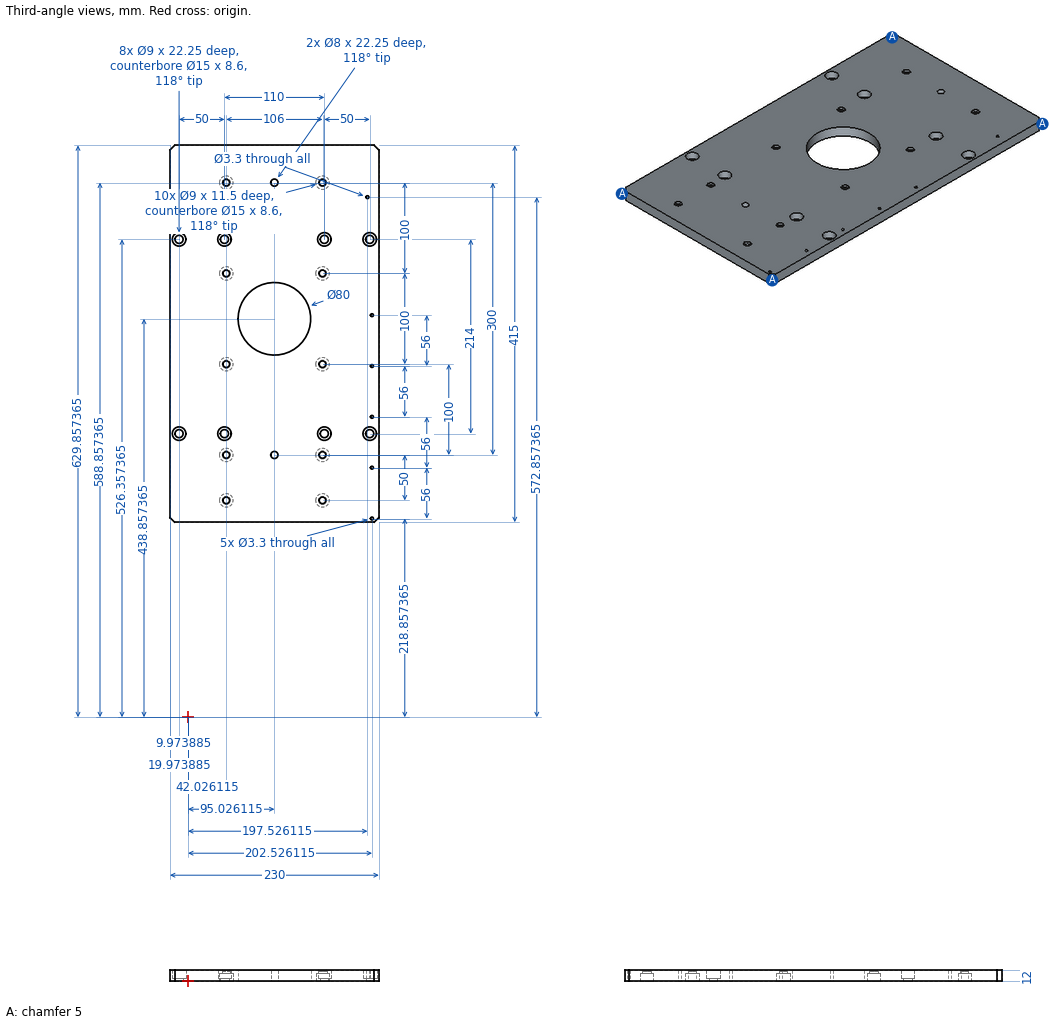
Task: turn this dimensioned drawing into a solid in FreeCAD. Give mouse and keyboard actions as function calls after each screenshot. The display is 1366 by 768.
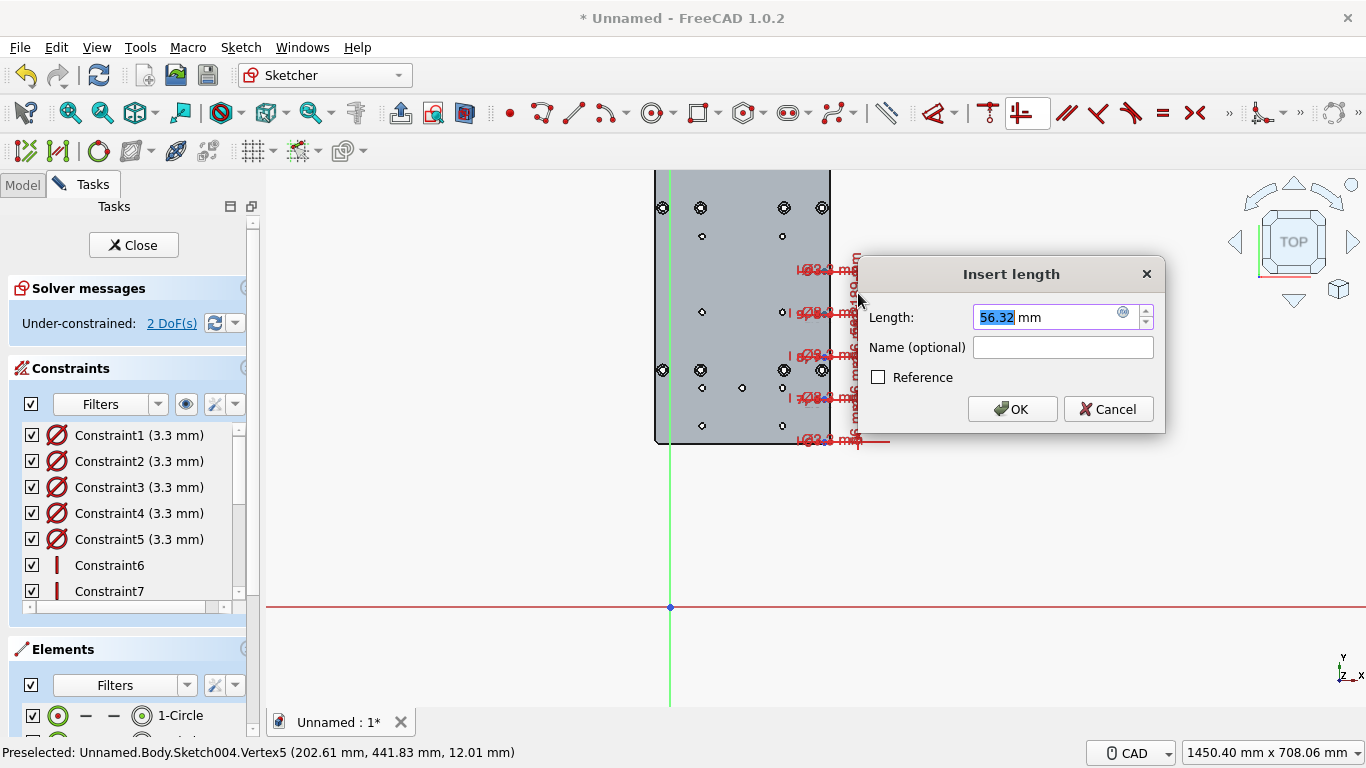
text(56)
key(Return)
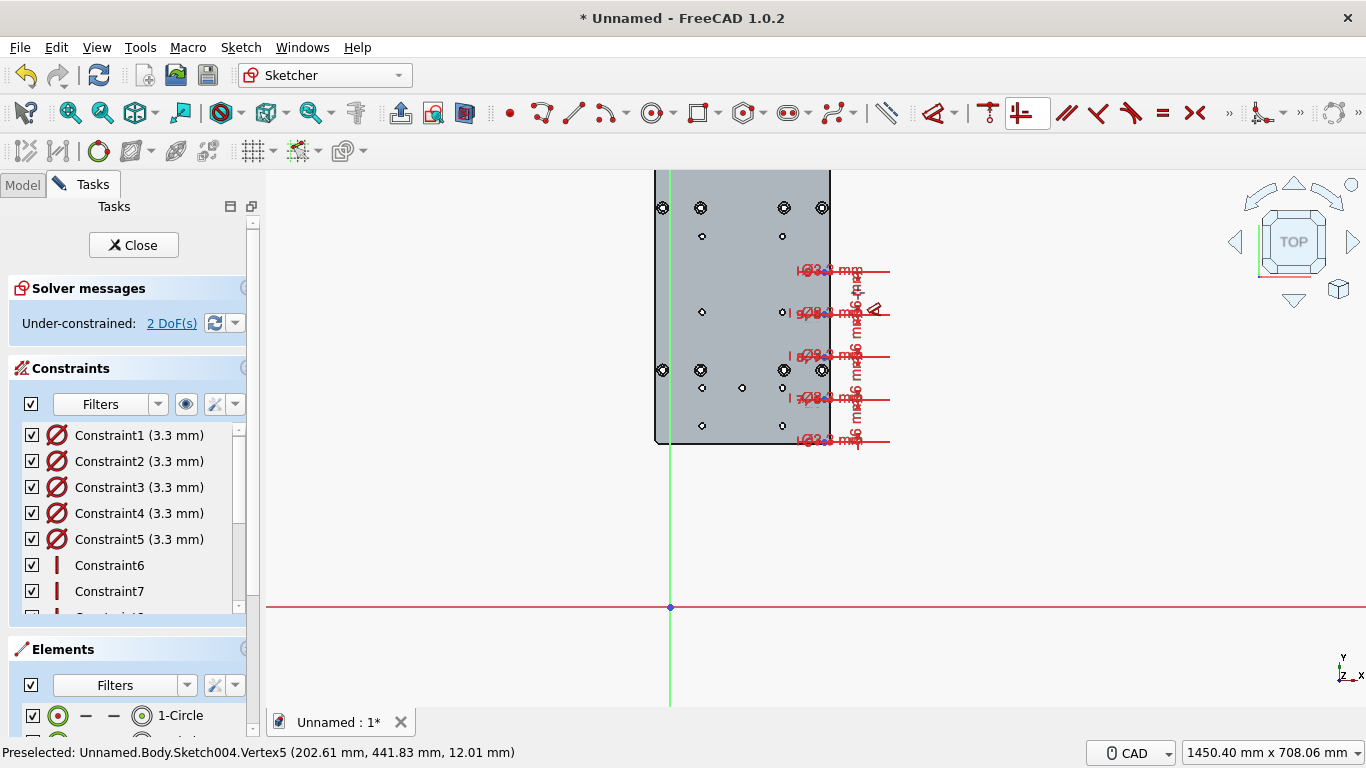
click(824, 442)
click(747, 641)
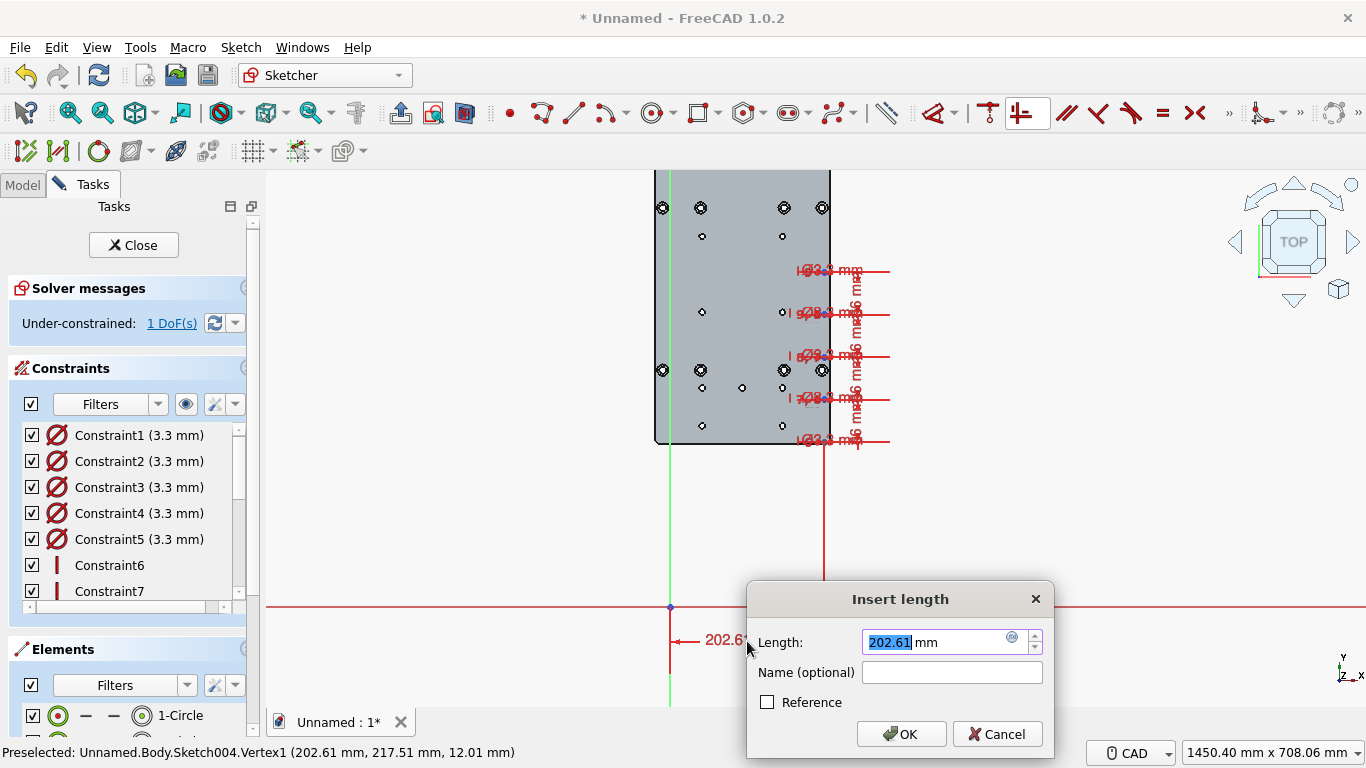
text(202.526115)
key(Return)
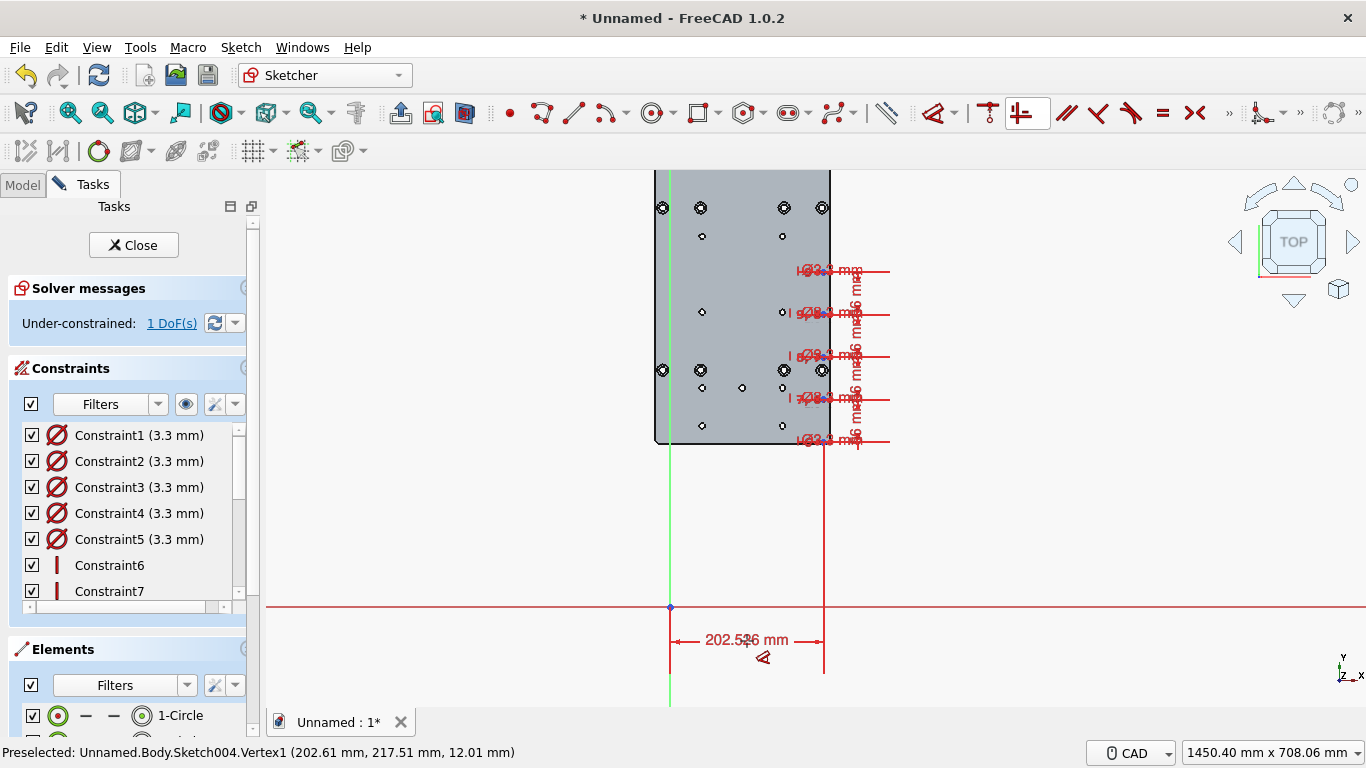
click(824, 442)
click(636, 525)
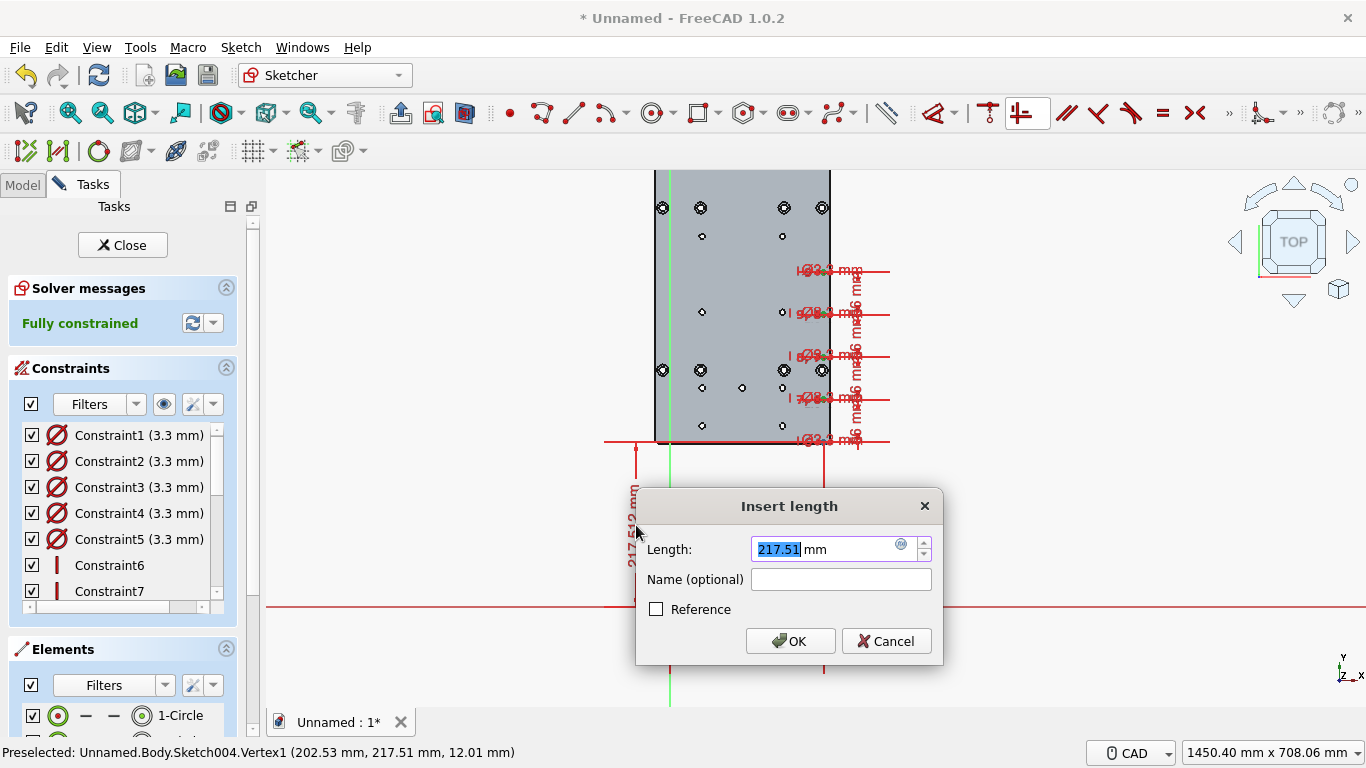
text(218.857365)
key(Return)
key(Escape)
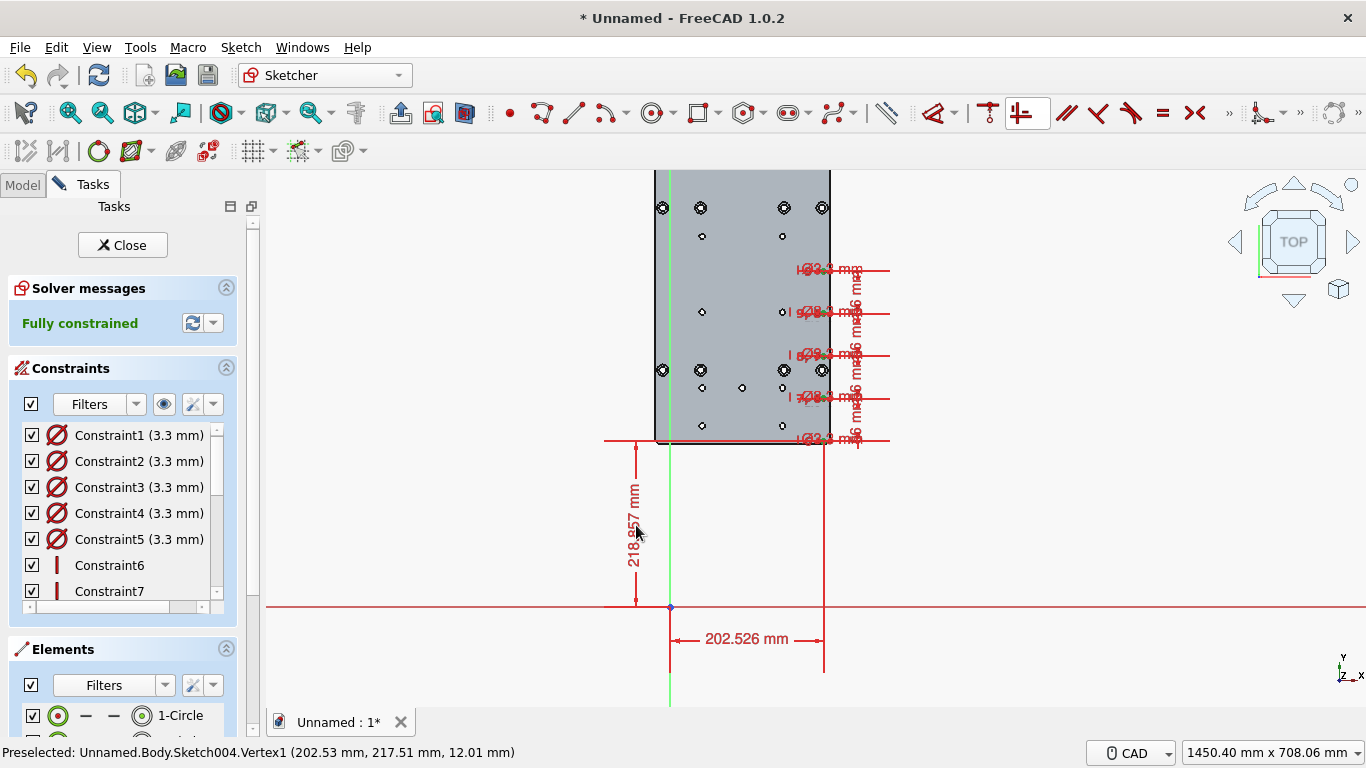
click(123, 245)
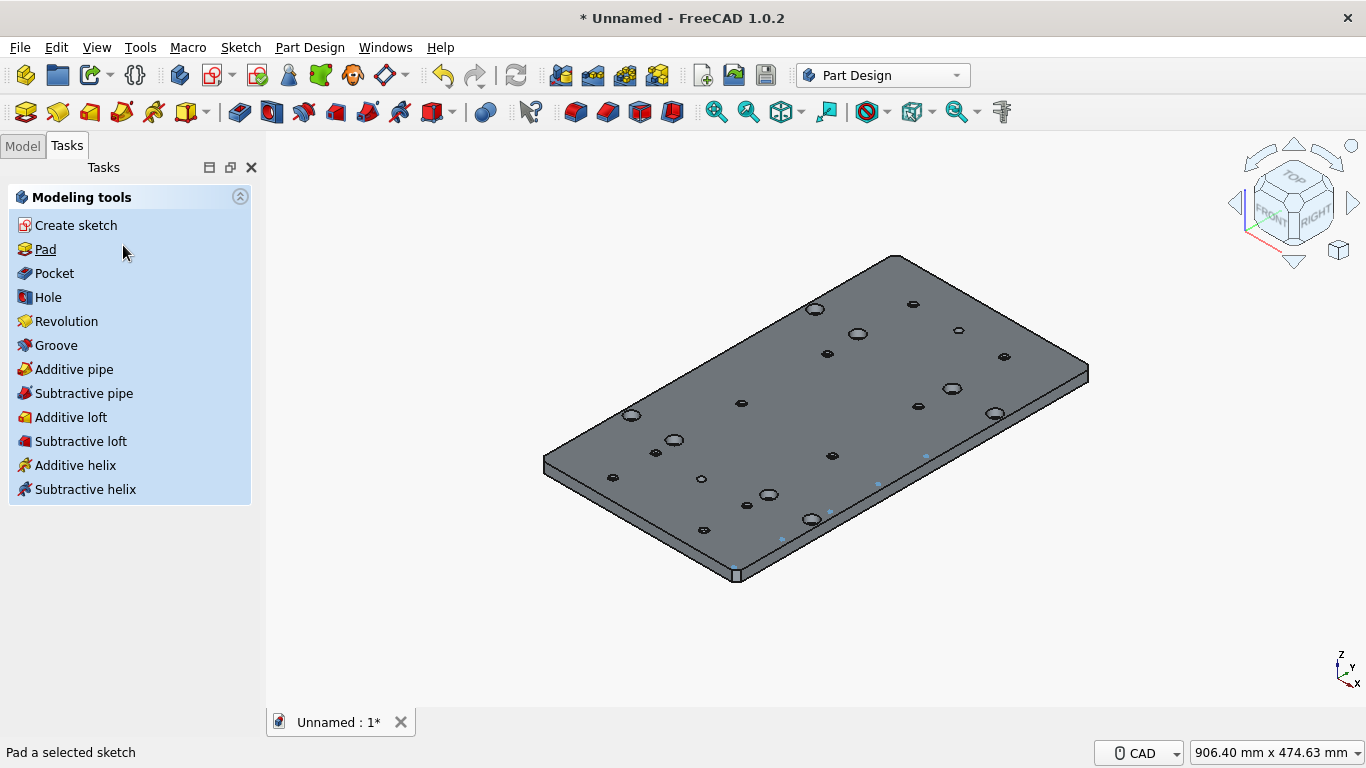
click(272, 112)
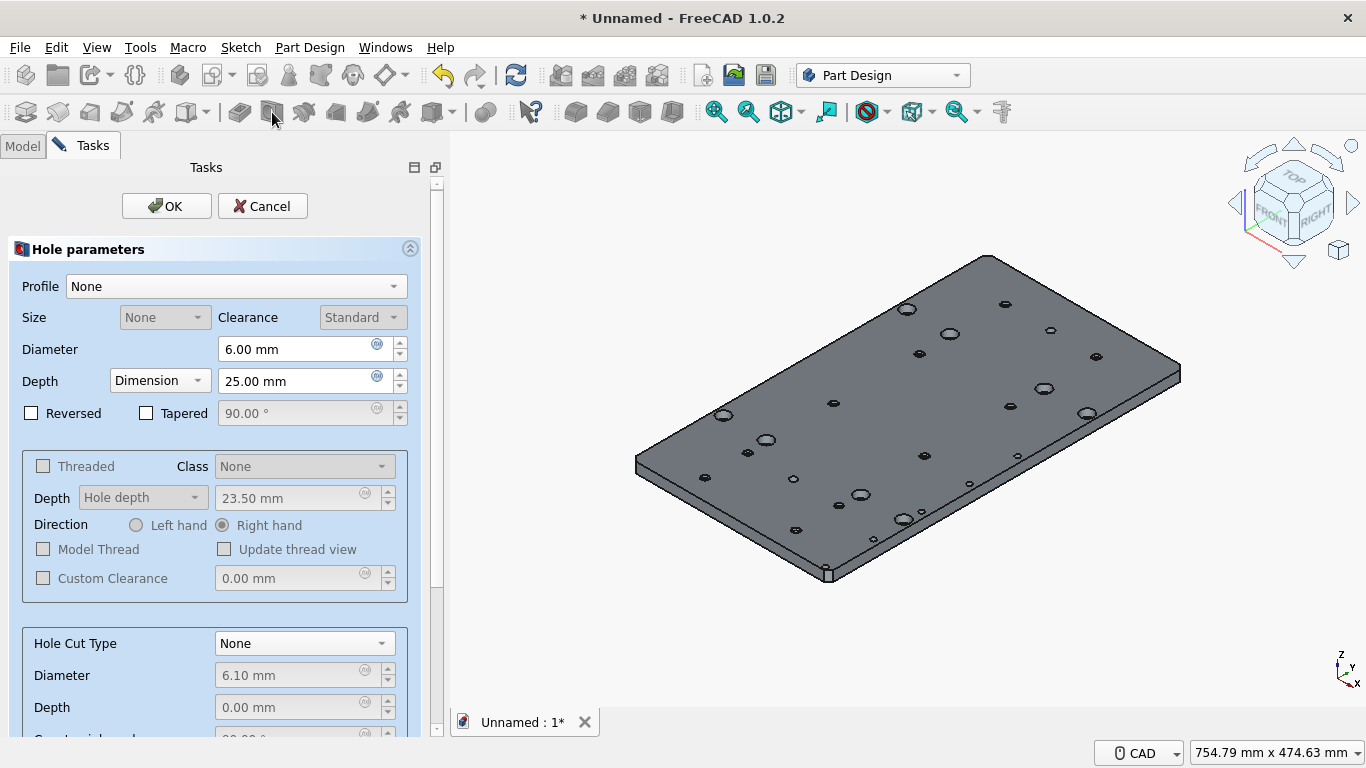
triple_click(305, 349)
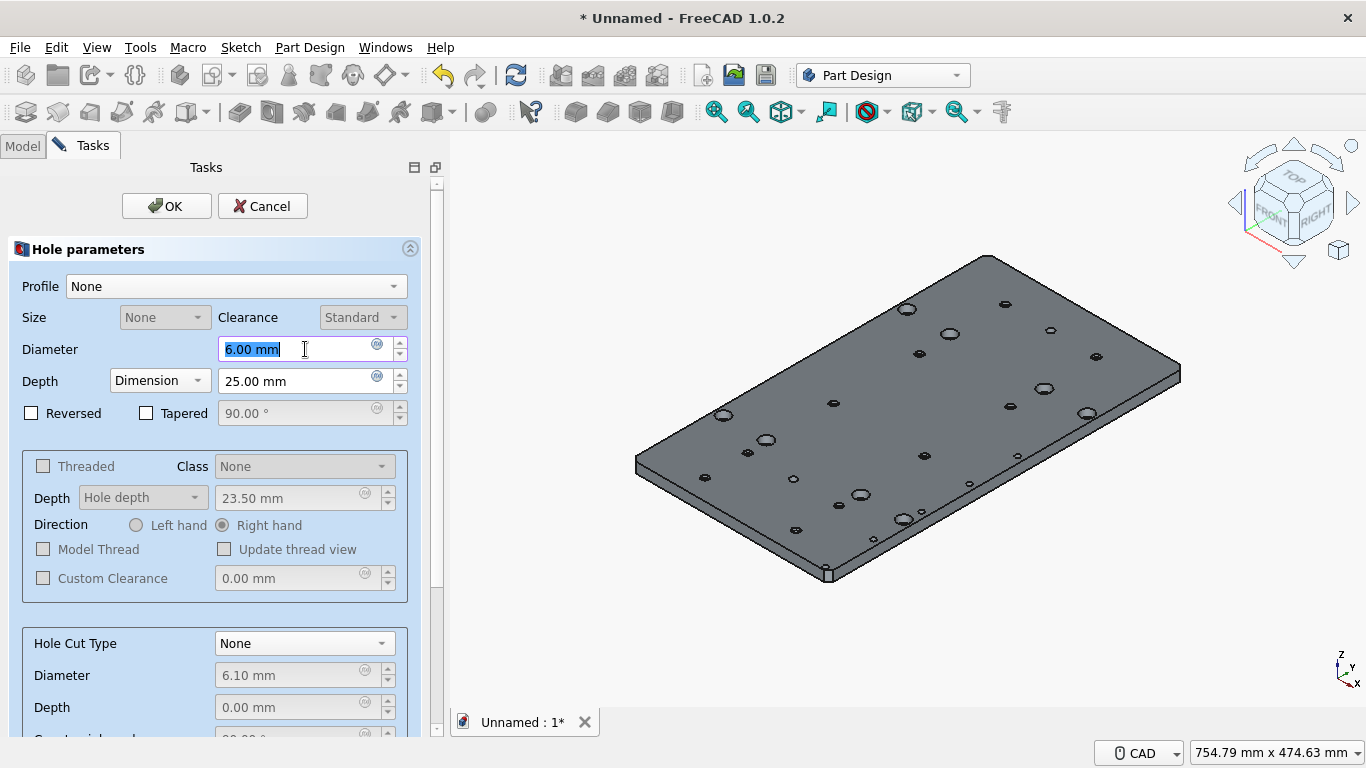
text(3.3)
key(Tab)